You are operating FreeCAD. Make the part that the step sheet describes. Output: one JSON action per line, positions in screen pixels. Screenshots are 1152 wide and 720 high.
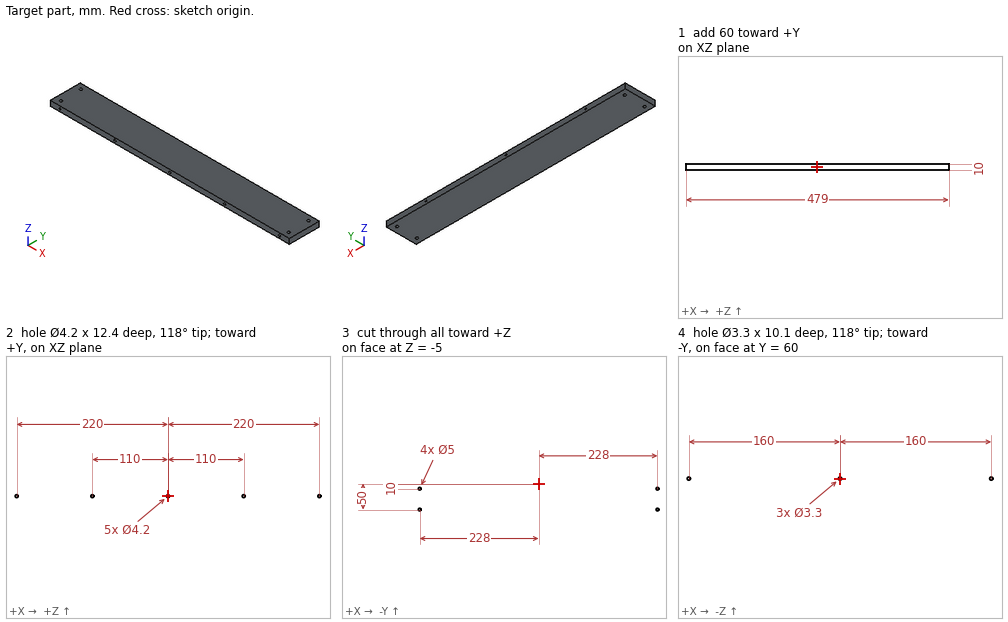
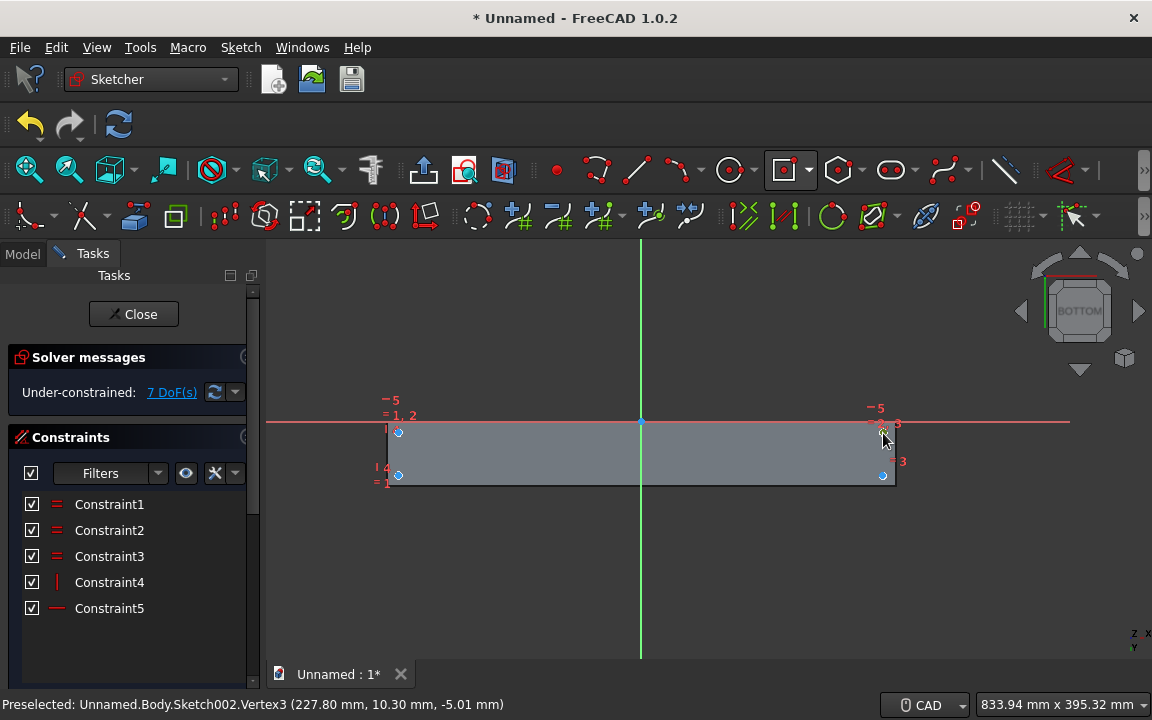
{"action": "left_click", "coordinate": [883, 476]}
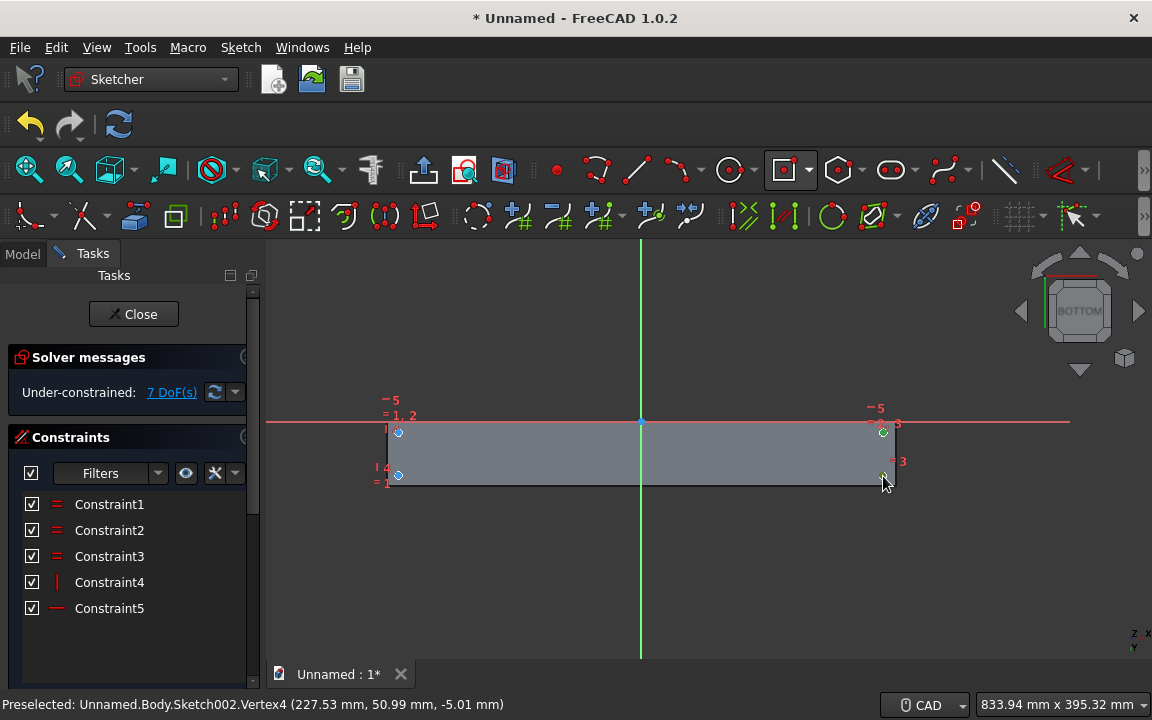
{"action": "key", "text": "v"}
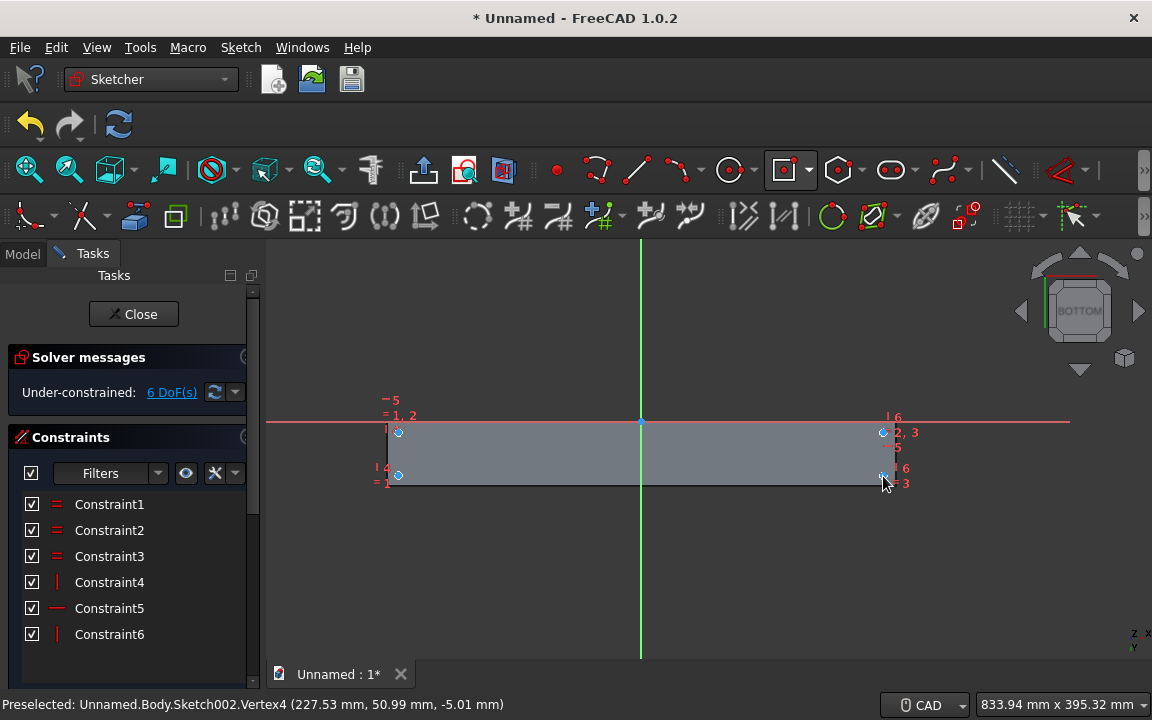
{"action": "left_click", "coordinate": [399, 476]}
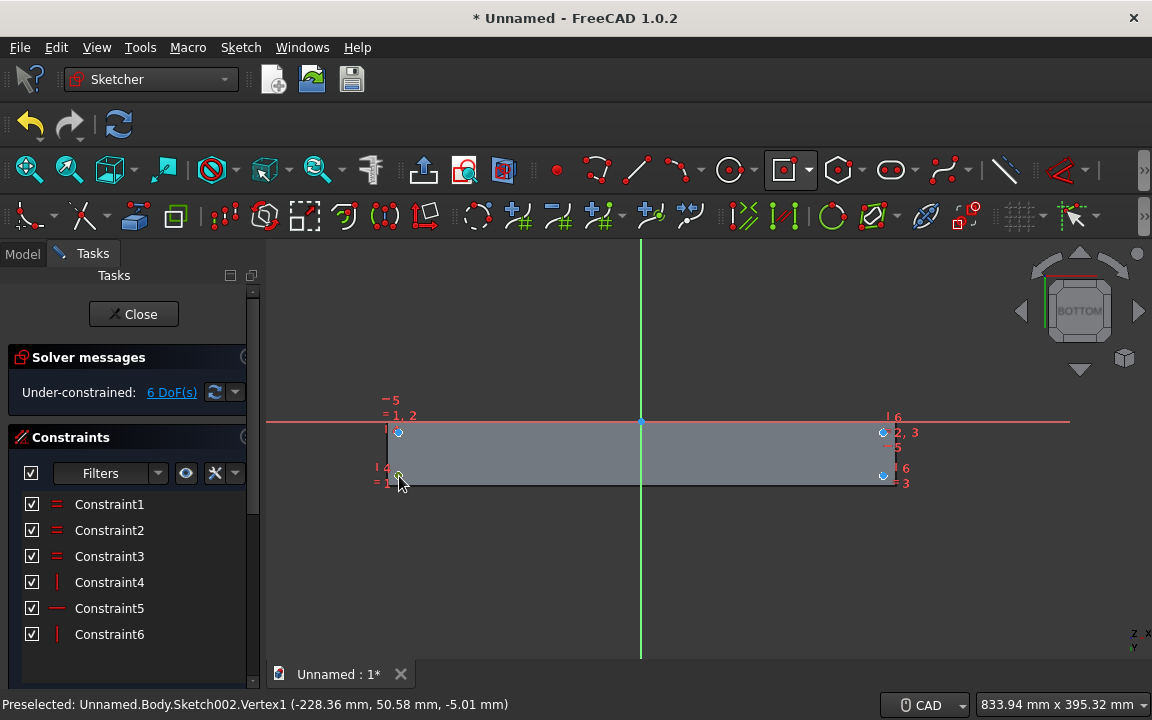
{"action": "left_click", "coordinate": [883, 476]}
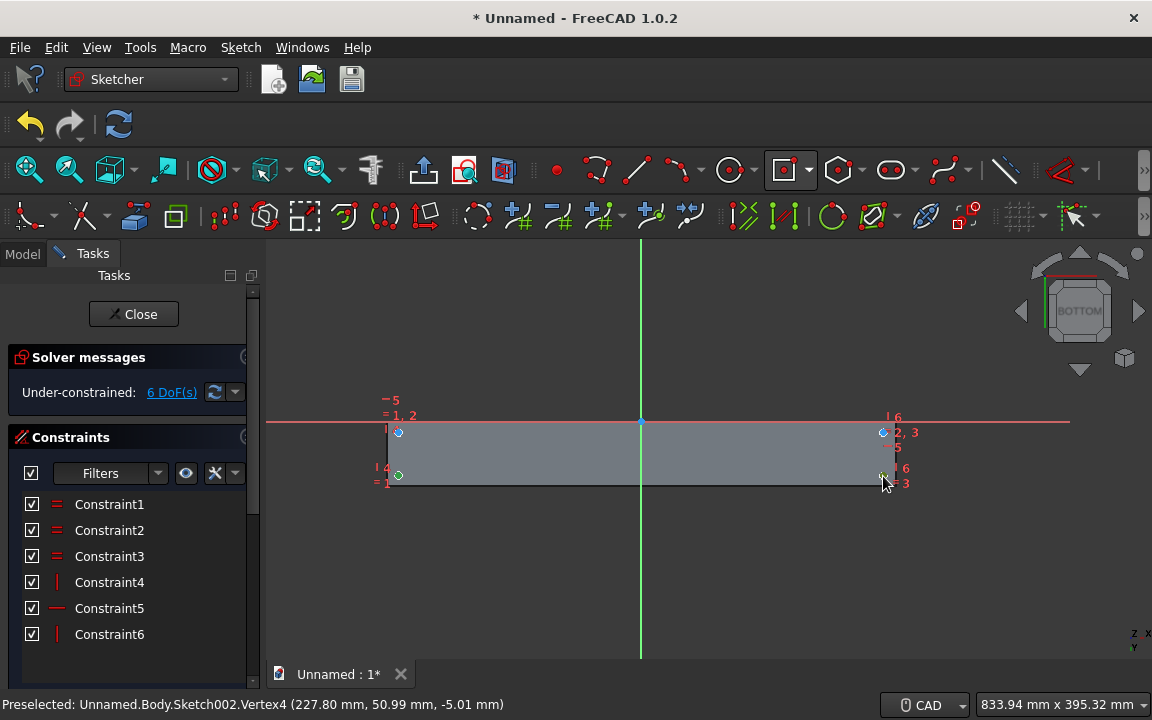
{"action": "key", "text": "h"}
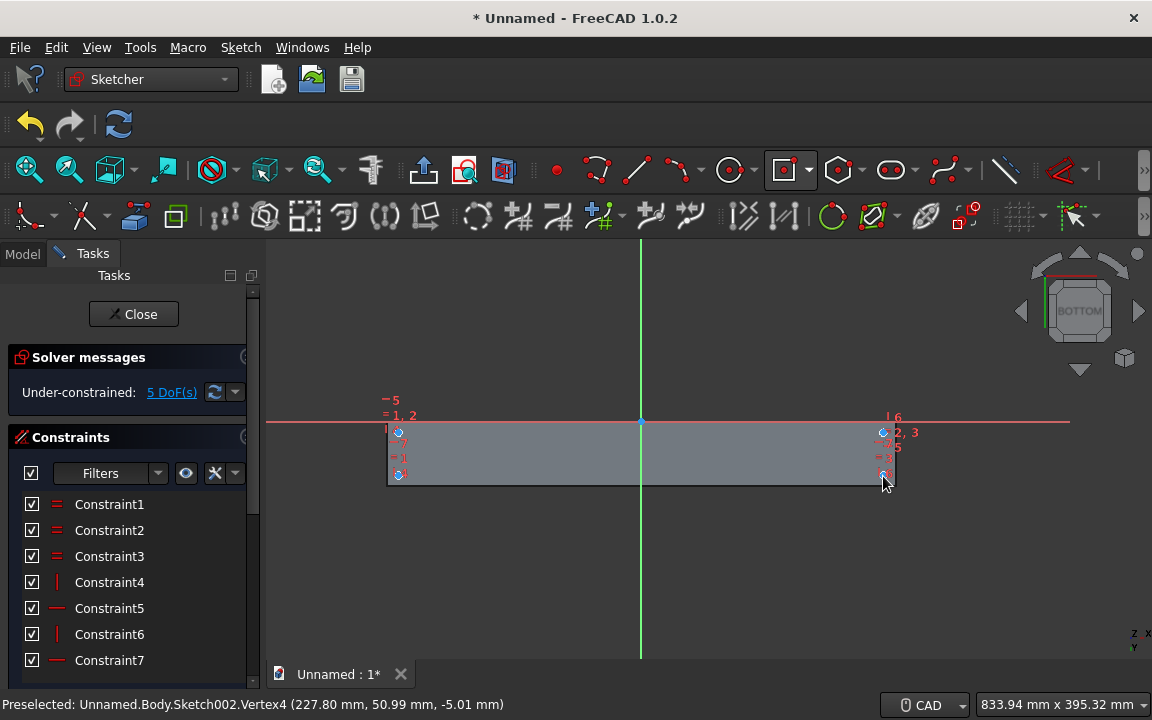
{"action": "key", "text": "d"}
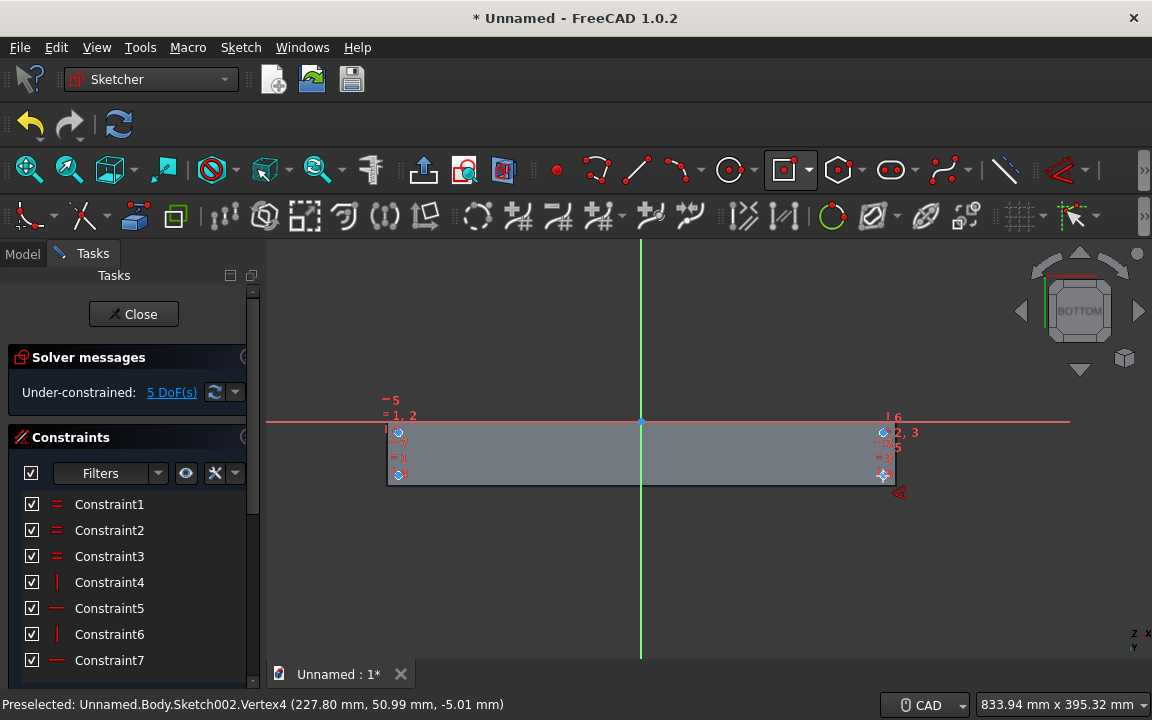
{"action": "scroll", "coordinate": [399, 479], "scroll_direction": "up", "scroll_amount": 11}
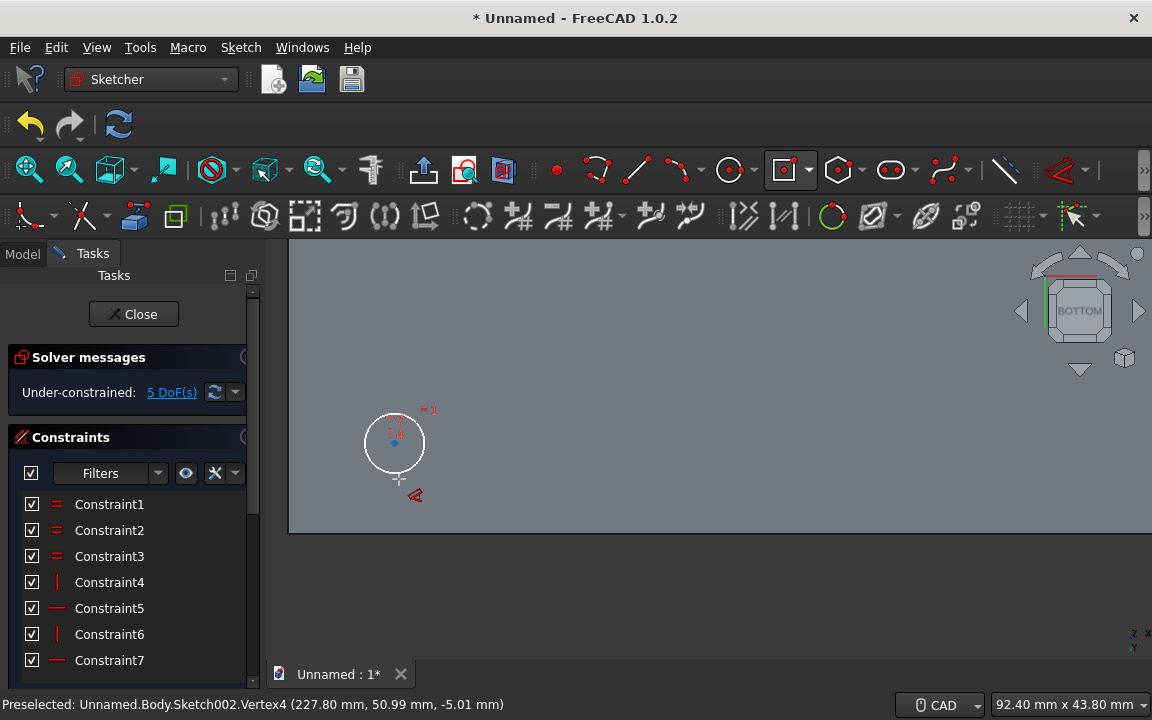
{"action": "left_click", "coordinate": [394, 473]}
{"action": "left_click", "coordinate": [393, 505]}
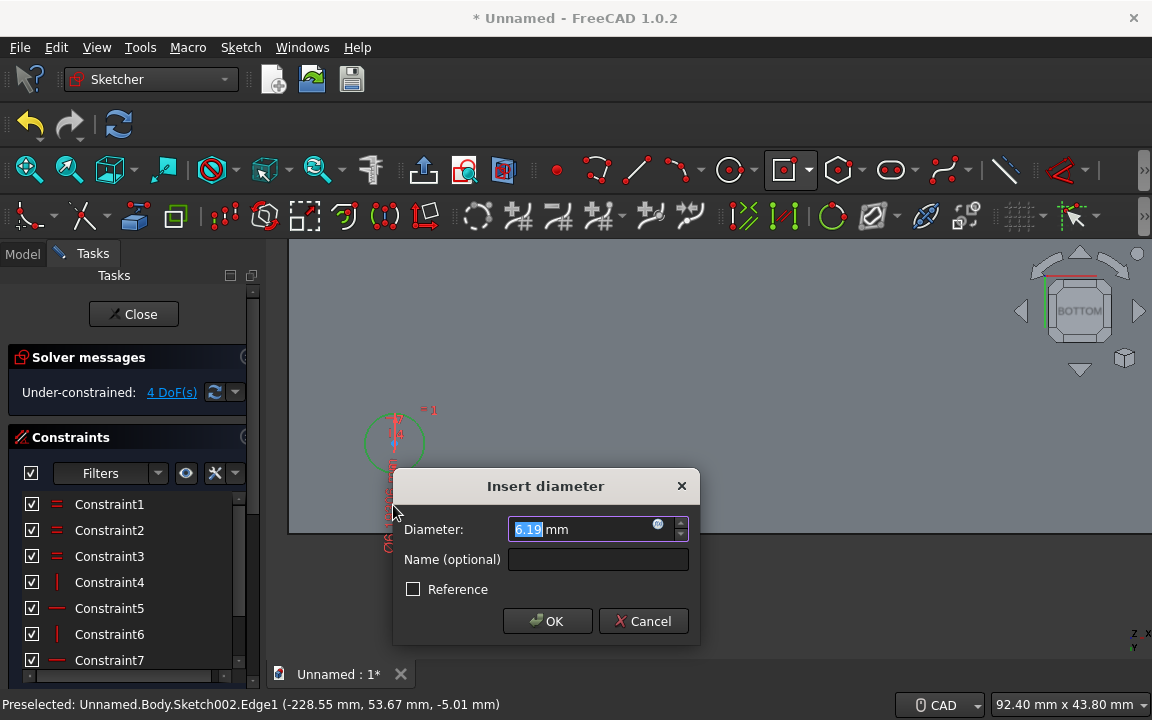
{"action": "type", "text": "5"}
{"action": "key", "text": "Return"}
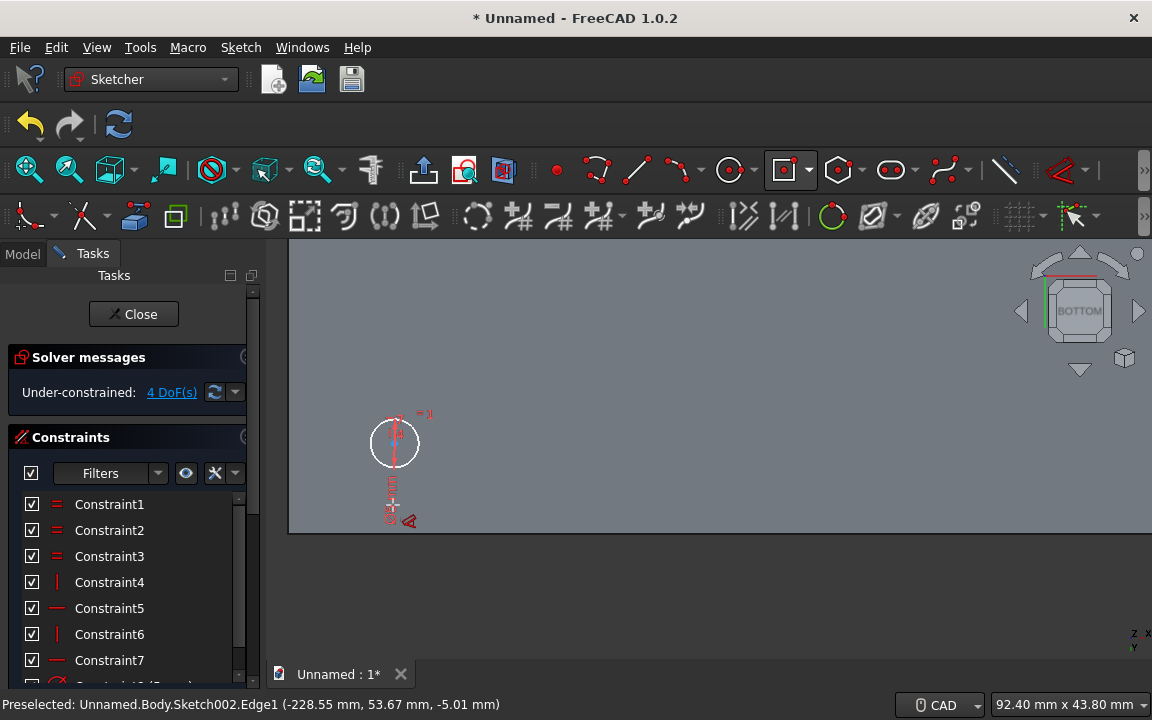
{"action": "scroll", "coordinate": [398, 479], "scroll_direction": "down", "scroll_amount": 11}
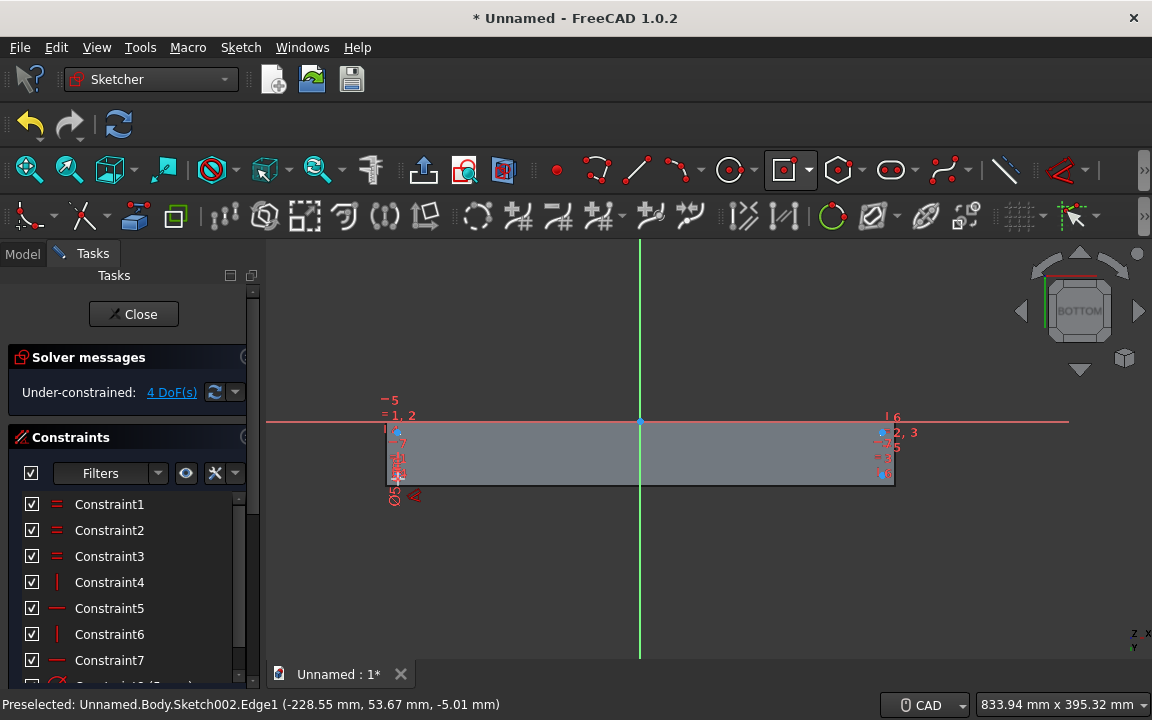
{"action": "left_click", "coordinate": [398, 476]}
{"action": "left_click", "coordinate": [364, 449]}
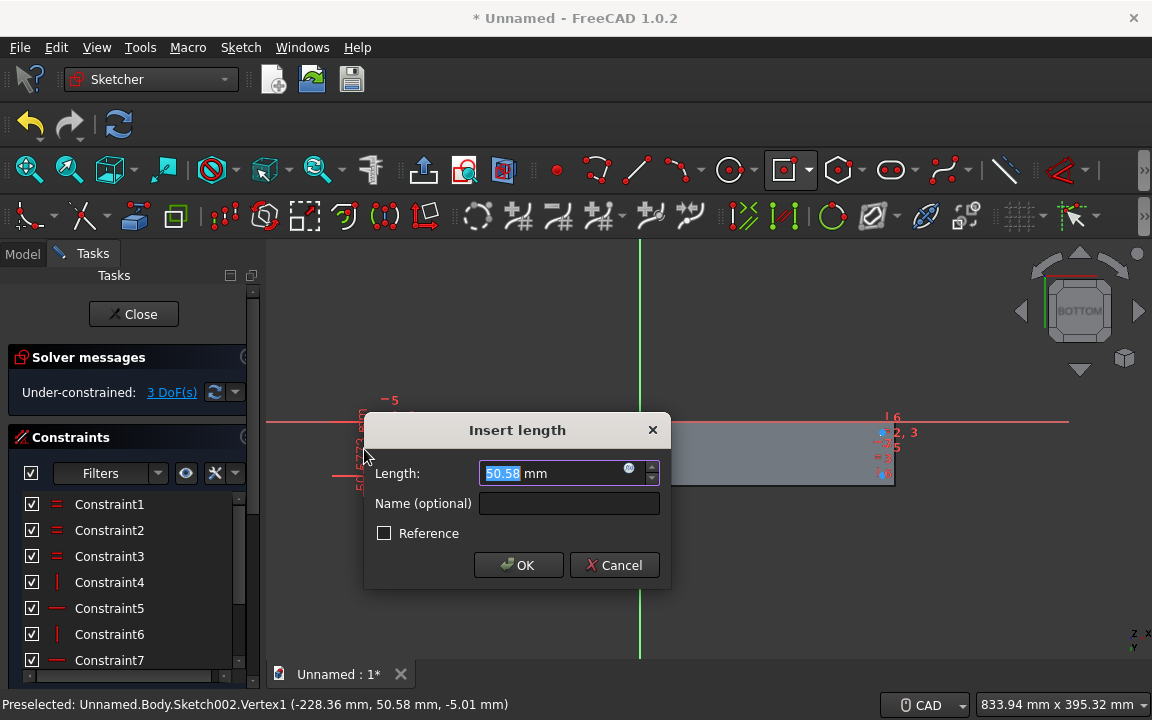
{"action": "type", "text": "50"}
{"action": "key", "text": "Return"}